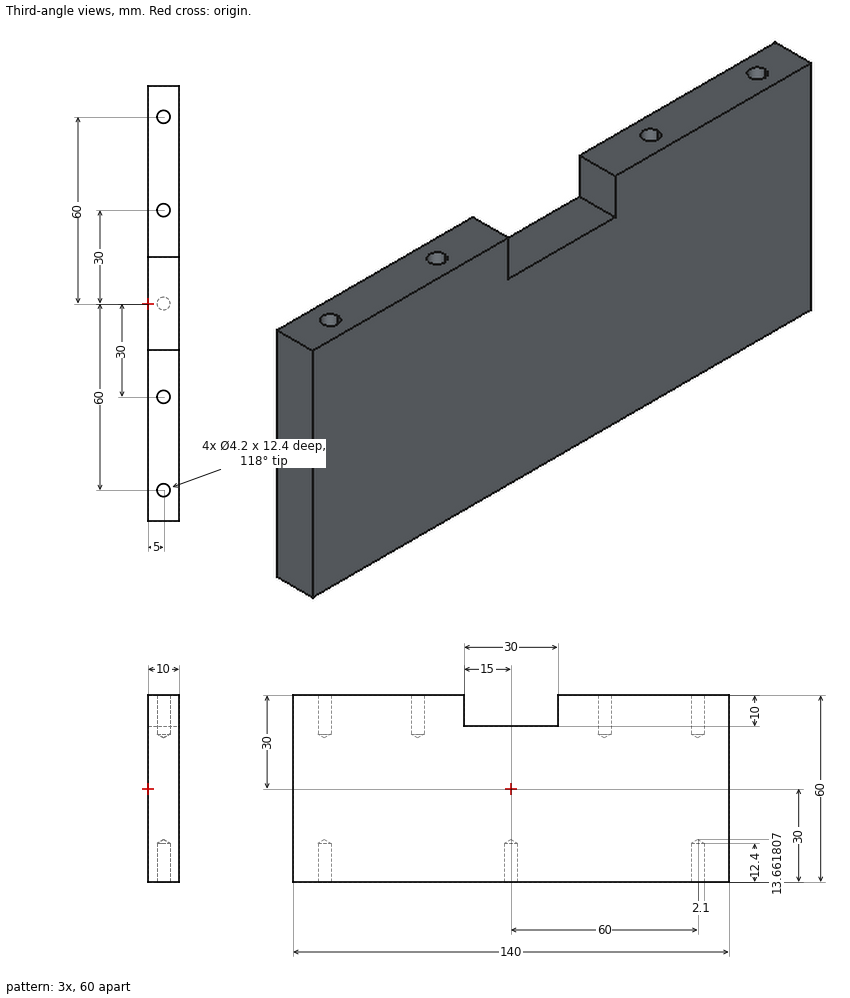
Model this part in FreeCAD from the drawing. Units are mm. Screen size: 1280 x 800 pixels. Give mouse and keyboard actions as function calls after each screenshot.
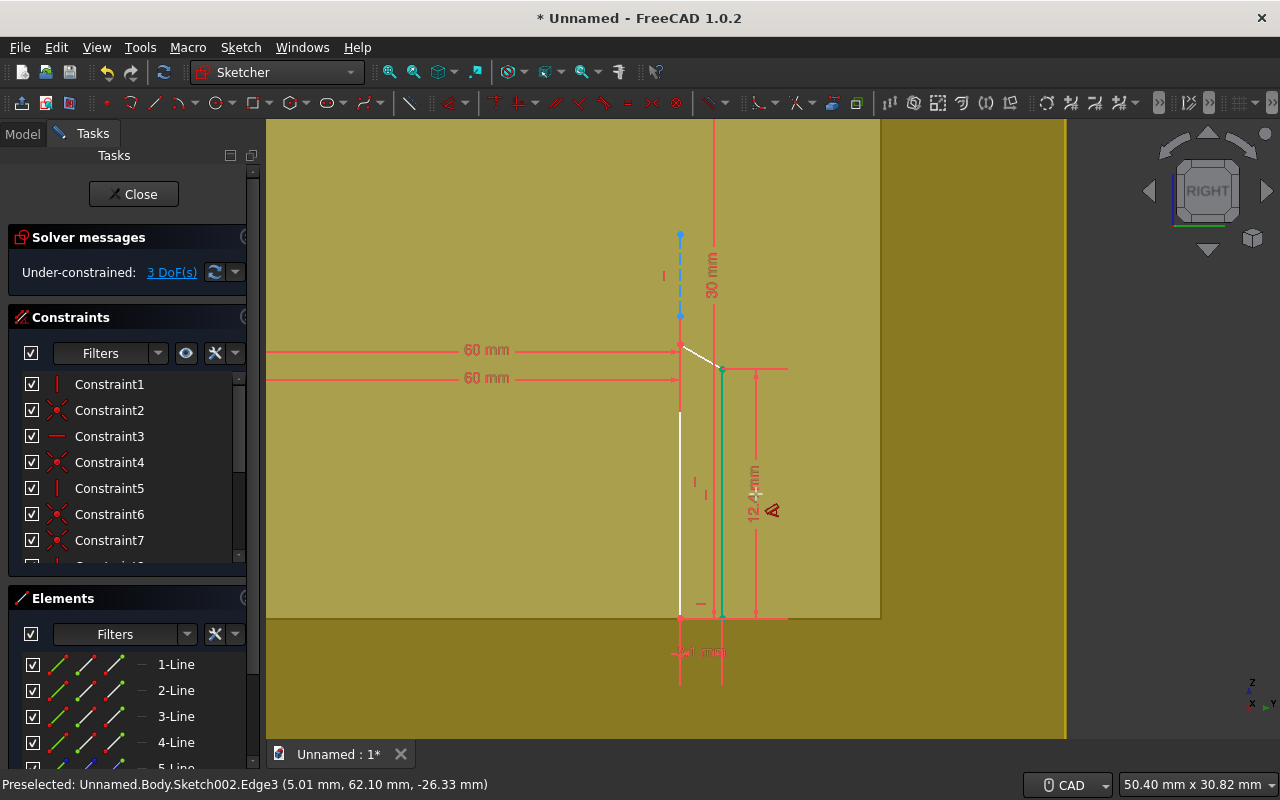
click(680, 427)
click(646, 482)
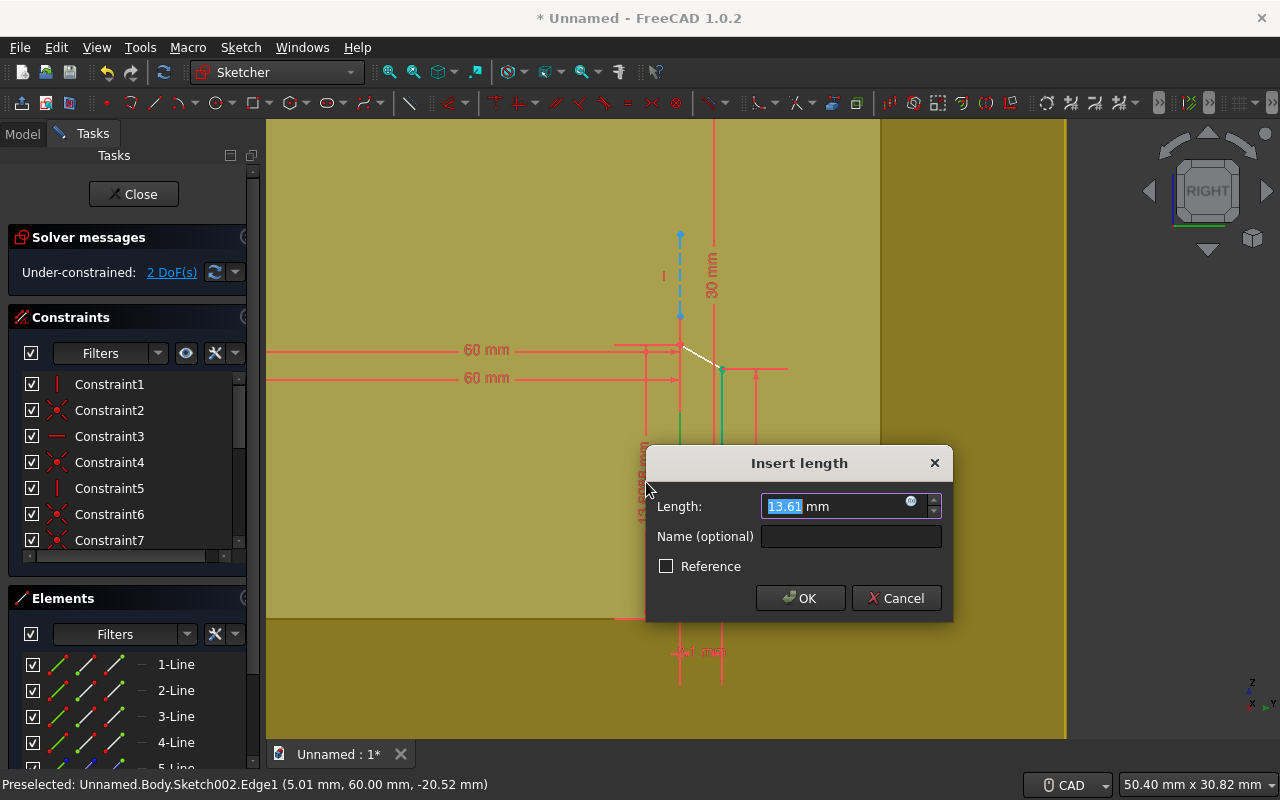
text(13.661807)
key(Return)
key(Escape)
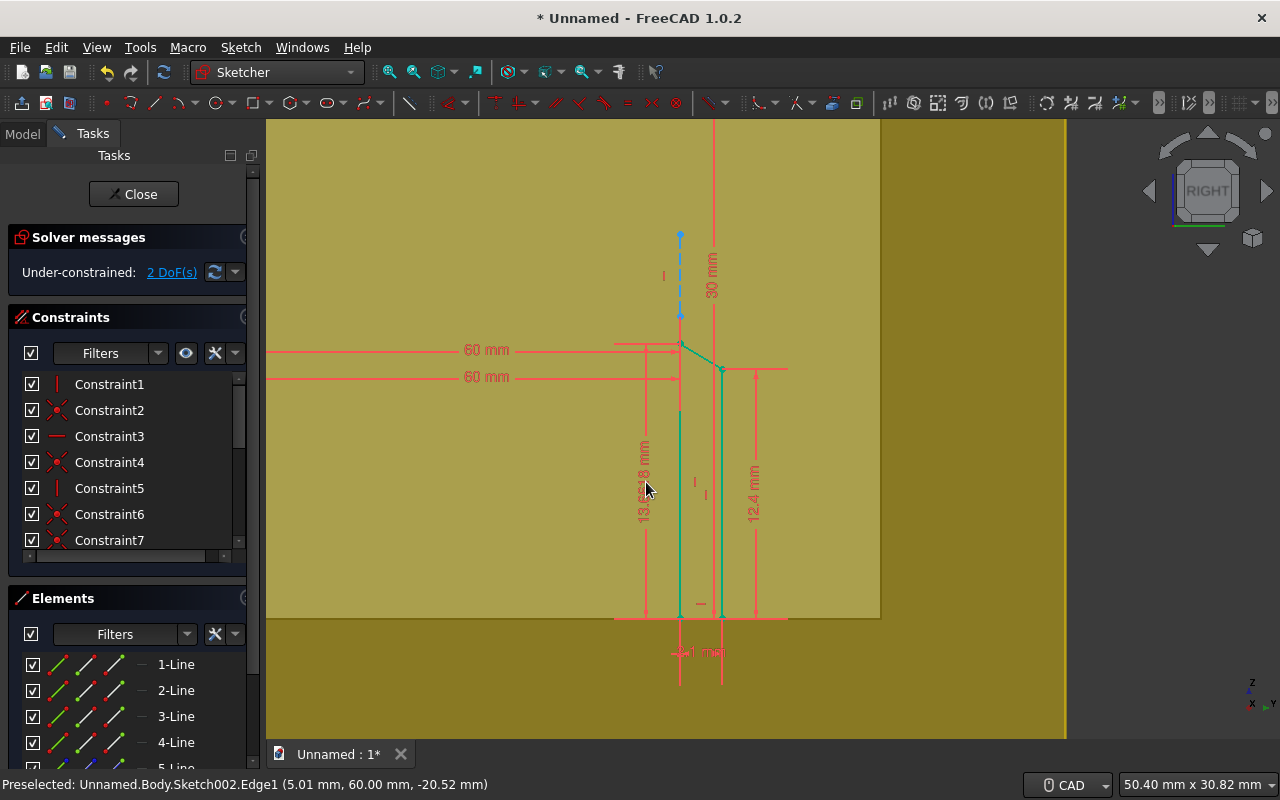
click(134, 194)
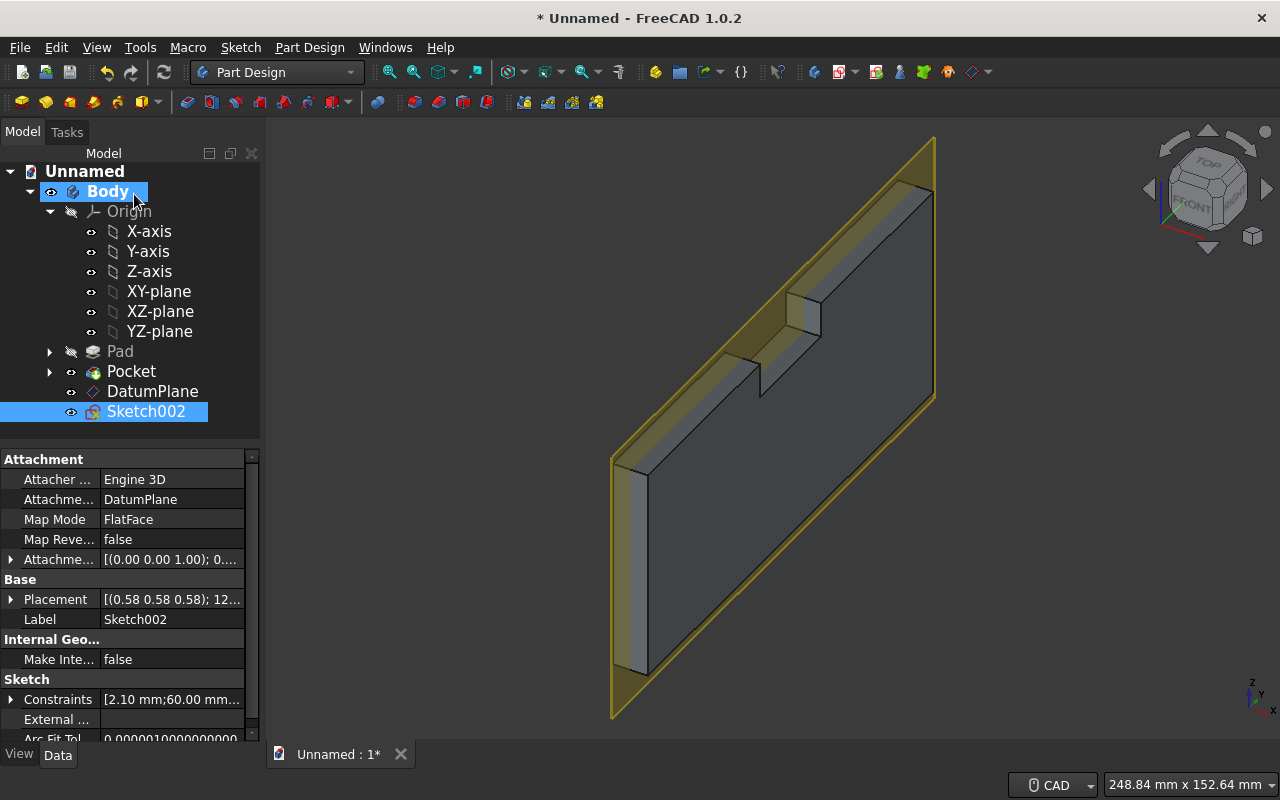
click(236, 102)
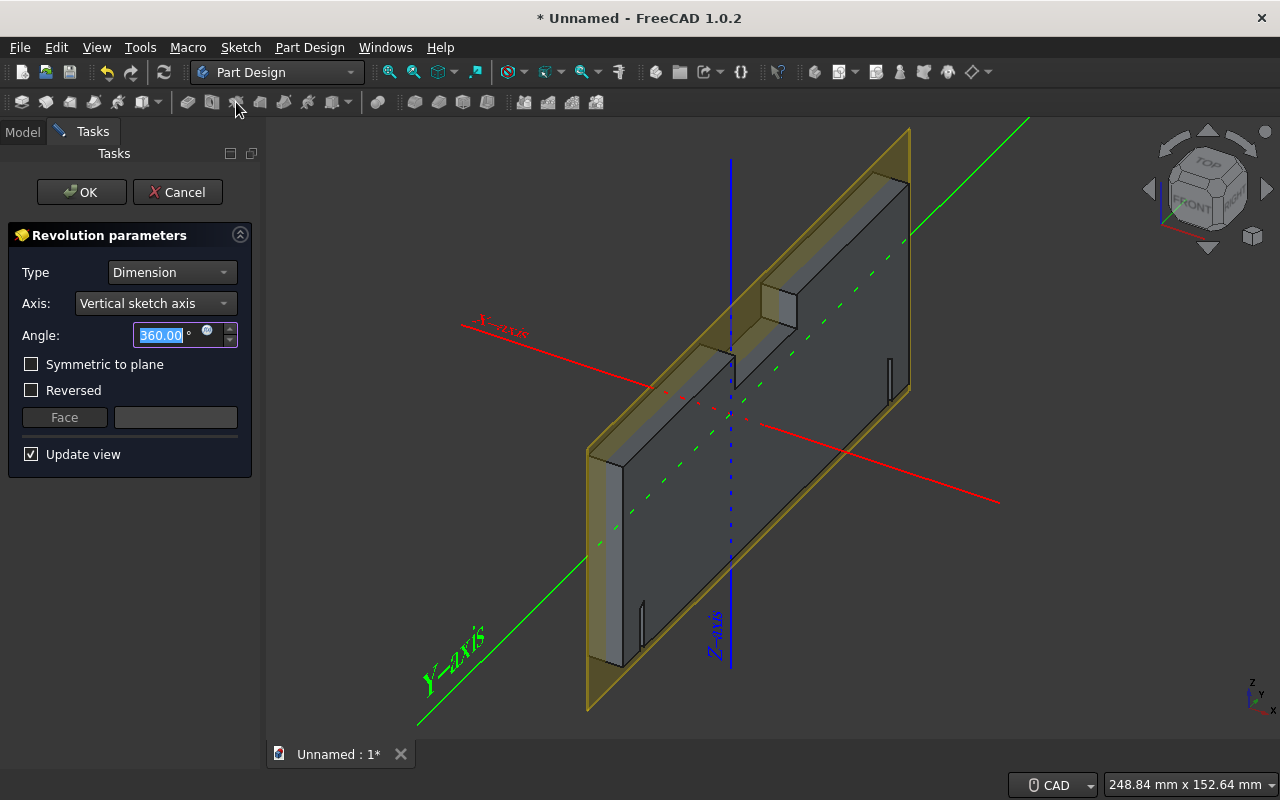
click(156, 304)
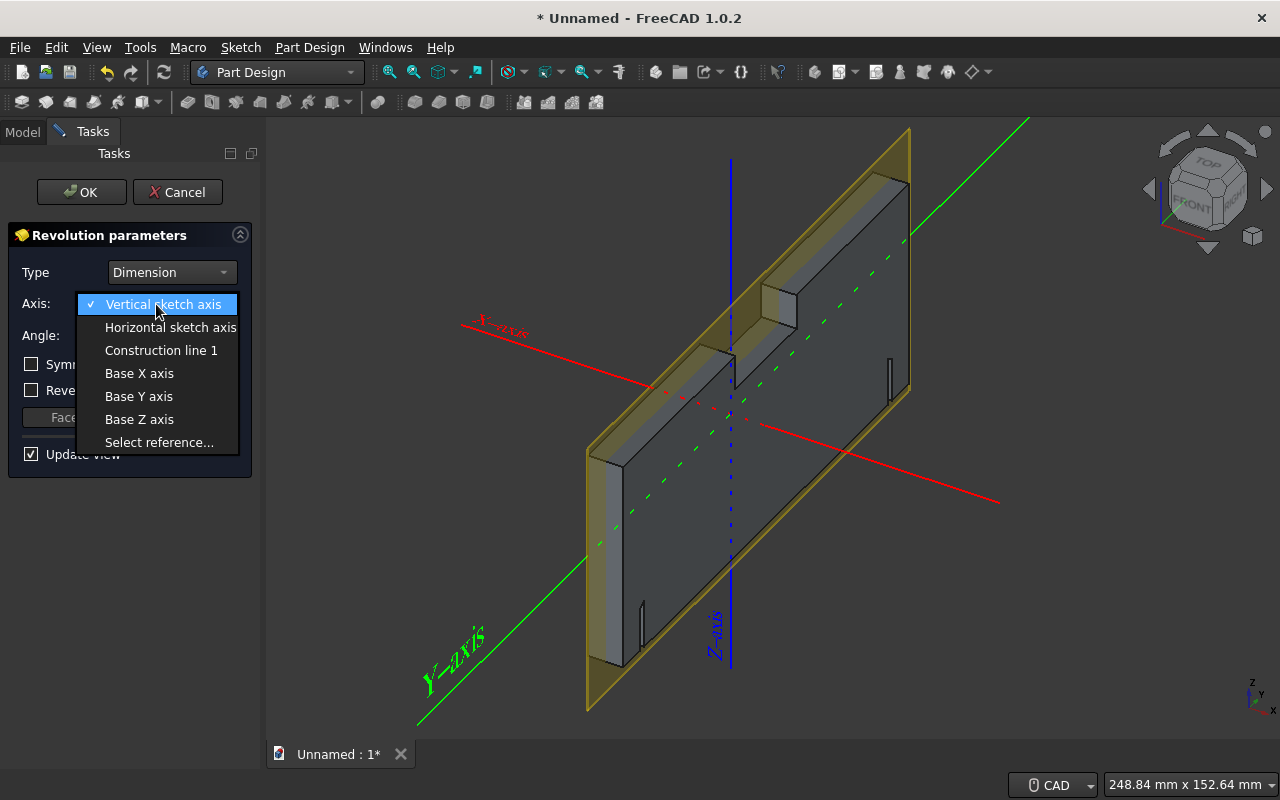
click(156, 350)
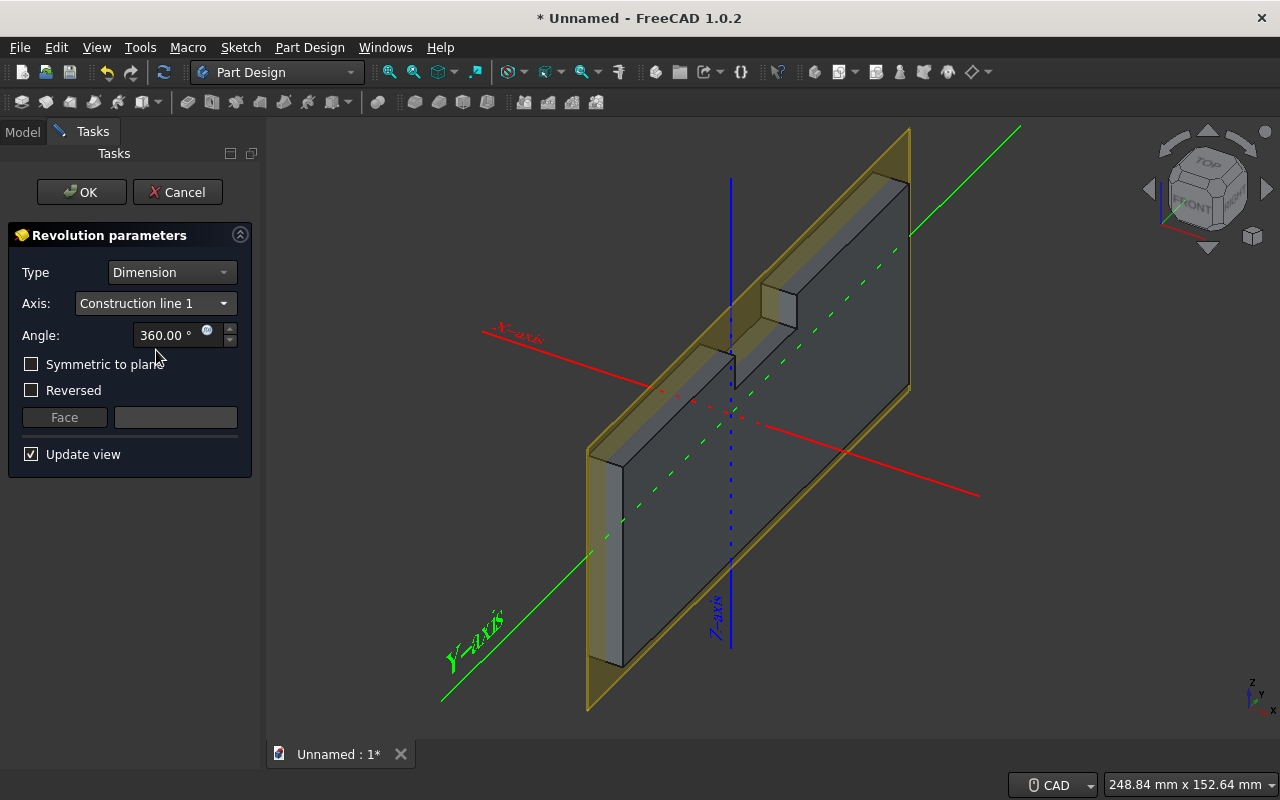
click(82, 192)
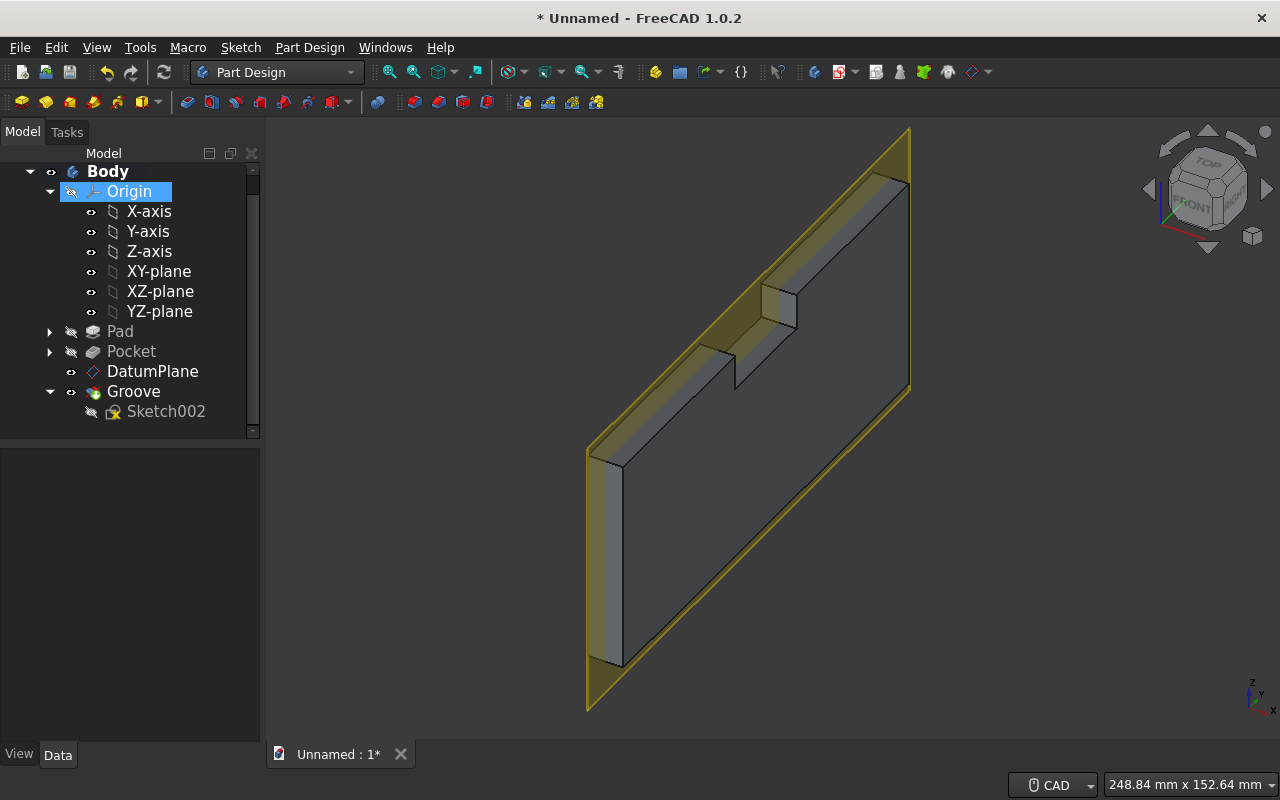
click(116, 372)
key(space)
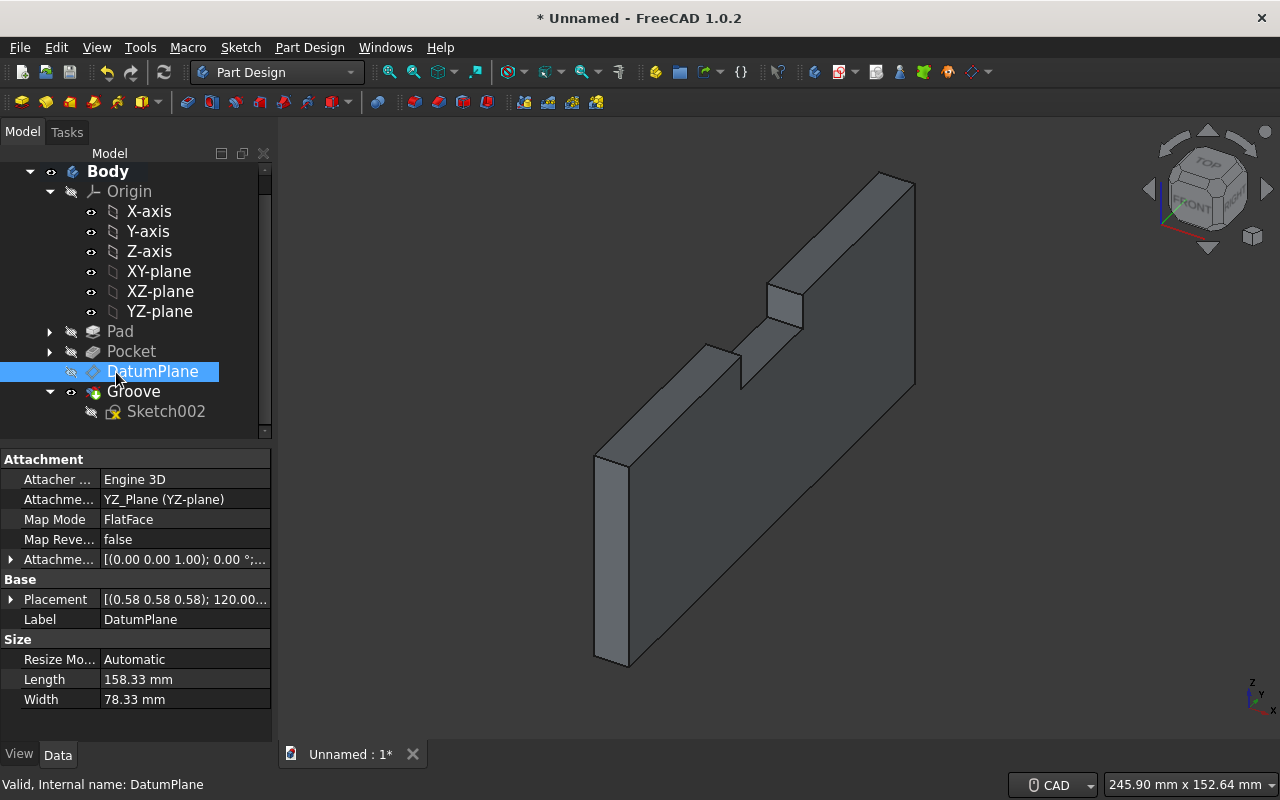
click(116, 392)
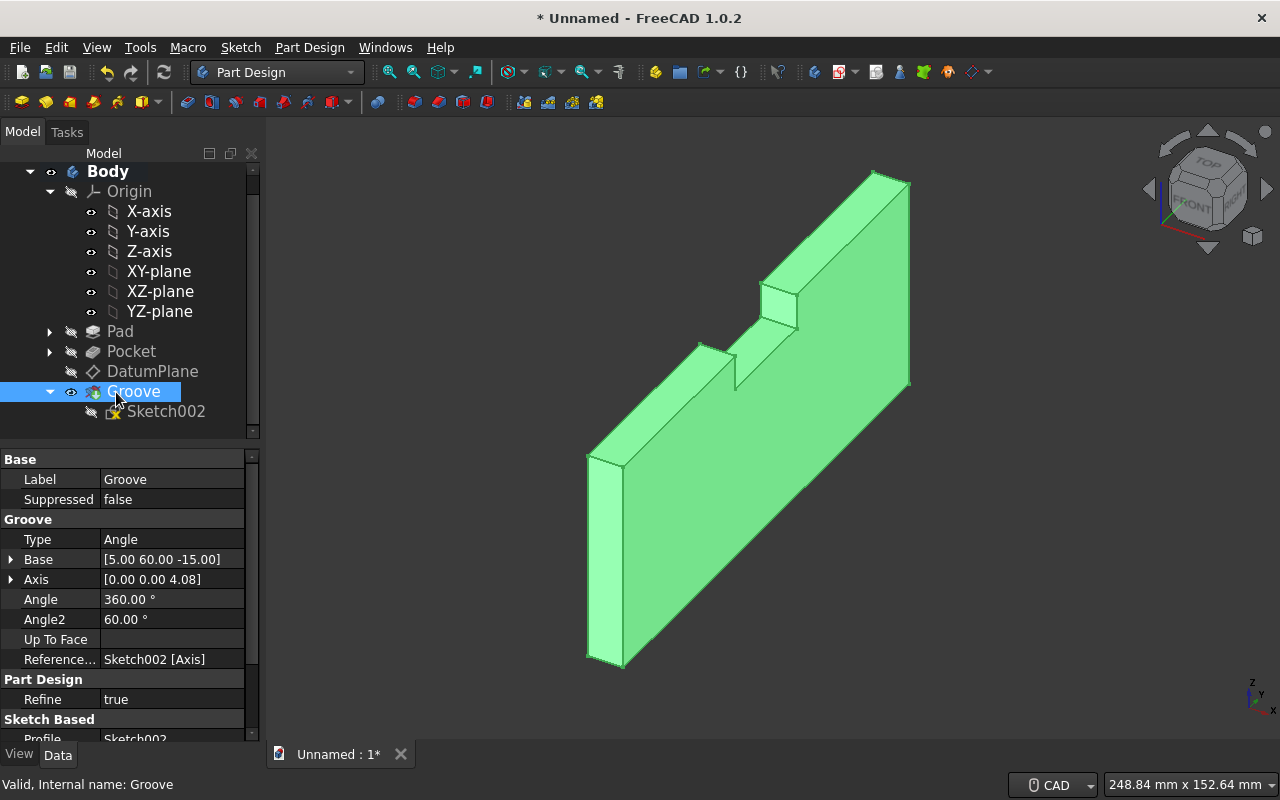
click(548, 102)